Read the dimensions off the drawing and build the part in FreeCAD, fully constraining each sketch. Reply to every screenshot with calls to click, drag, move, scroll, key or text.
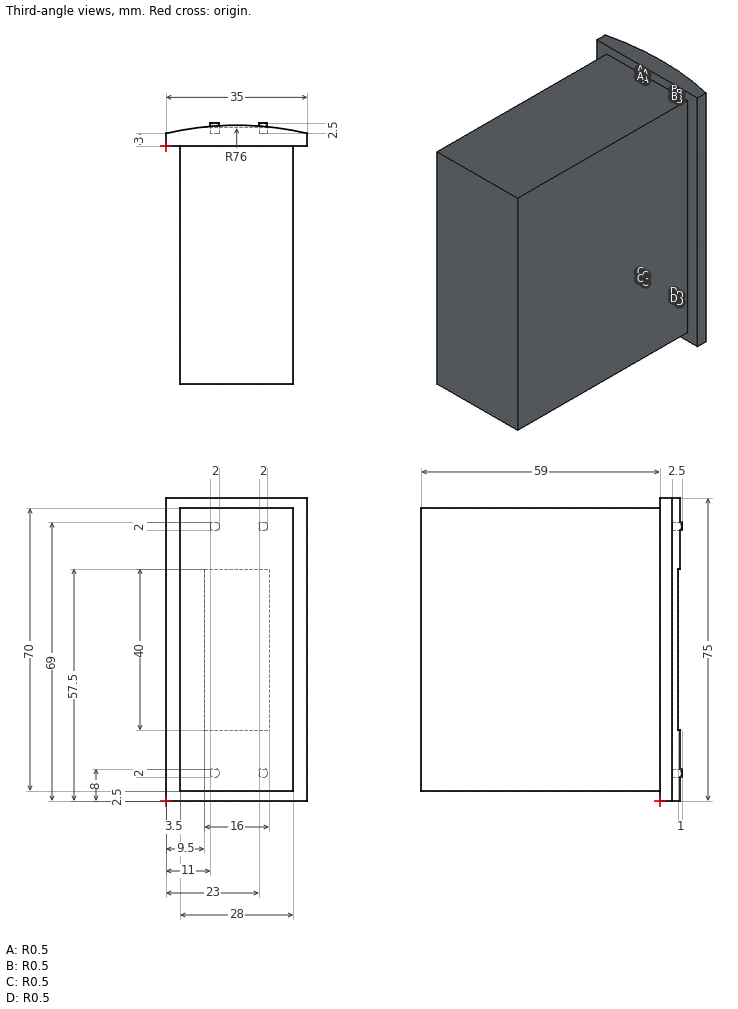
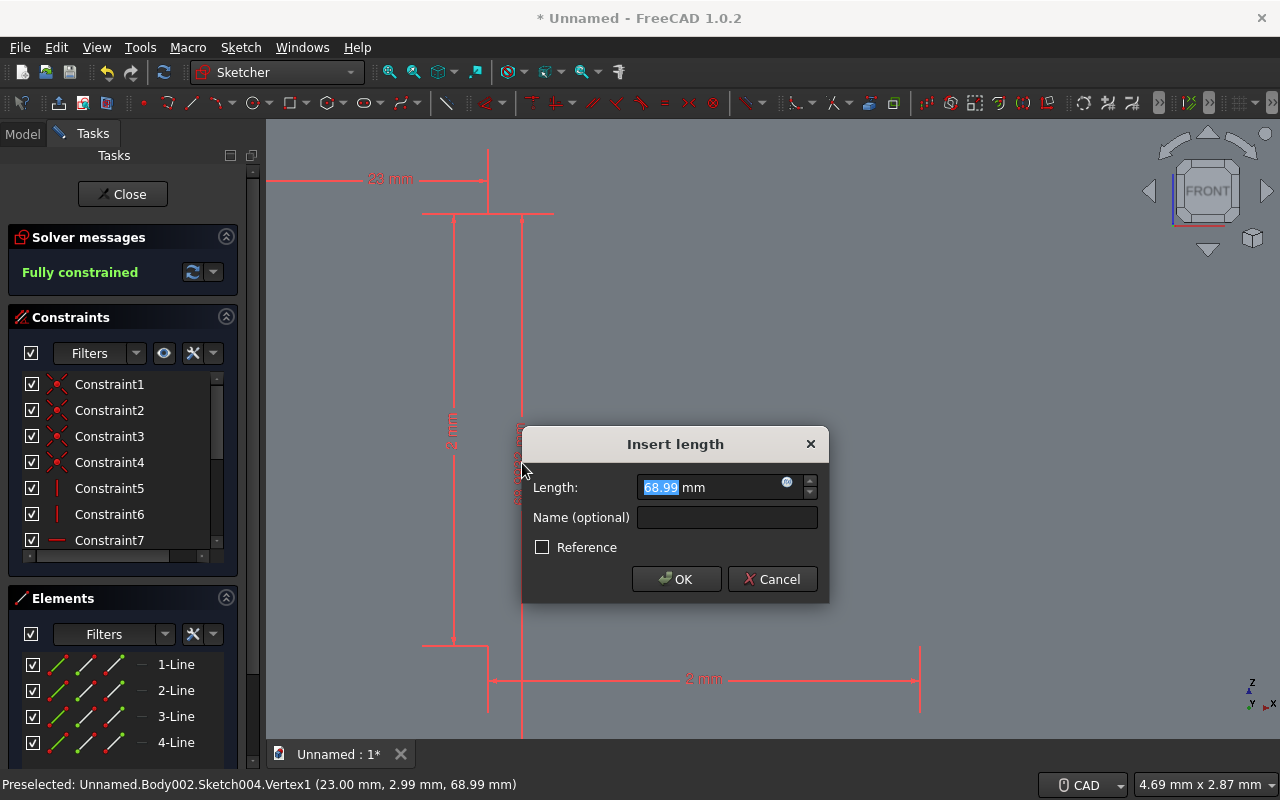
text(69)
key(Return)
key(Escape)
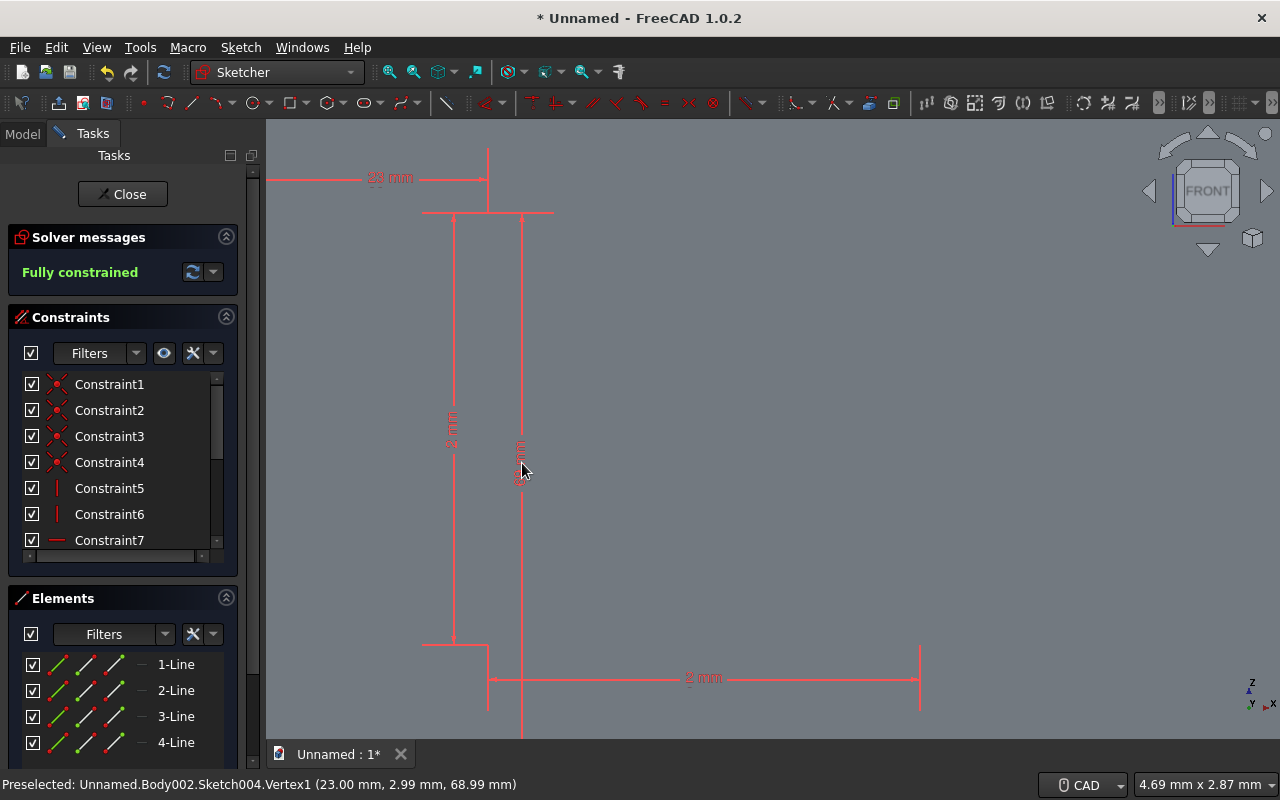
click(123, 194)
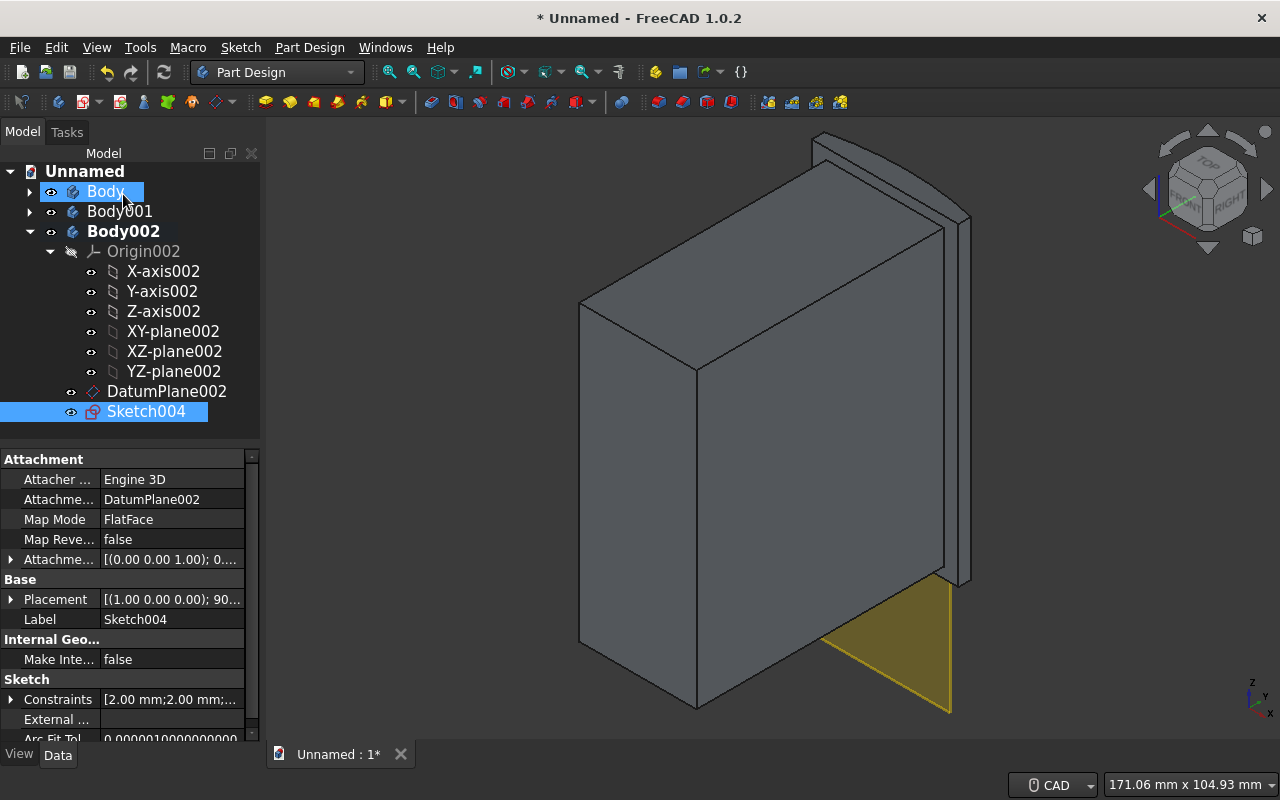
click(266, 102)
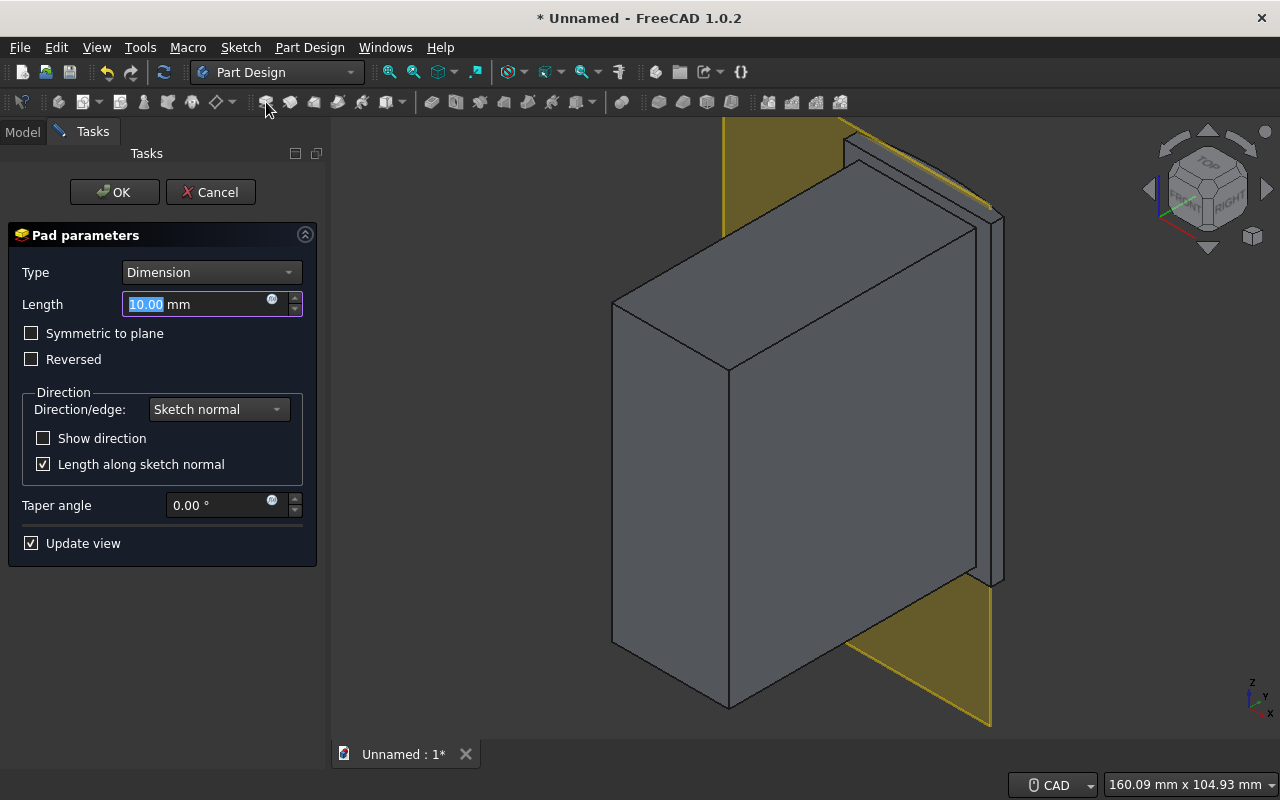
text(2.5)
key(Tab)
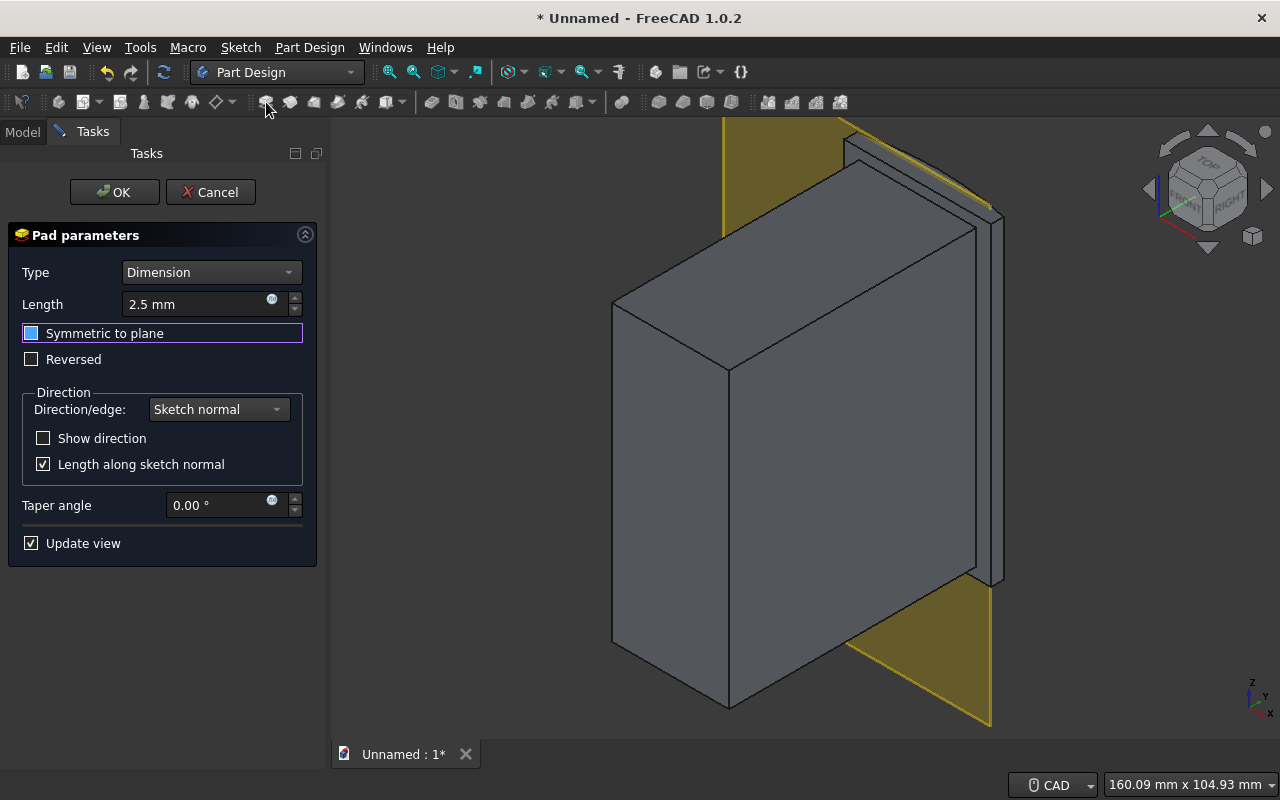
click(30, 359)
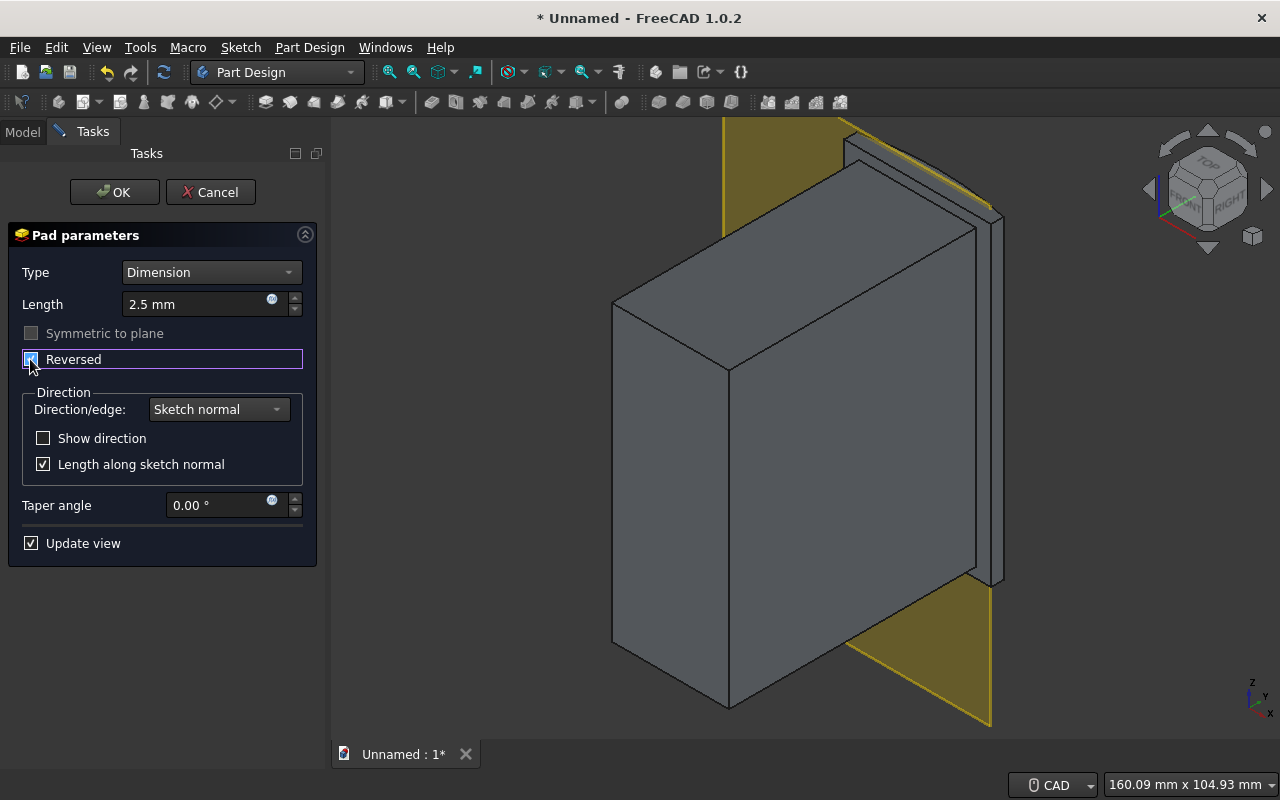
click(115, 192)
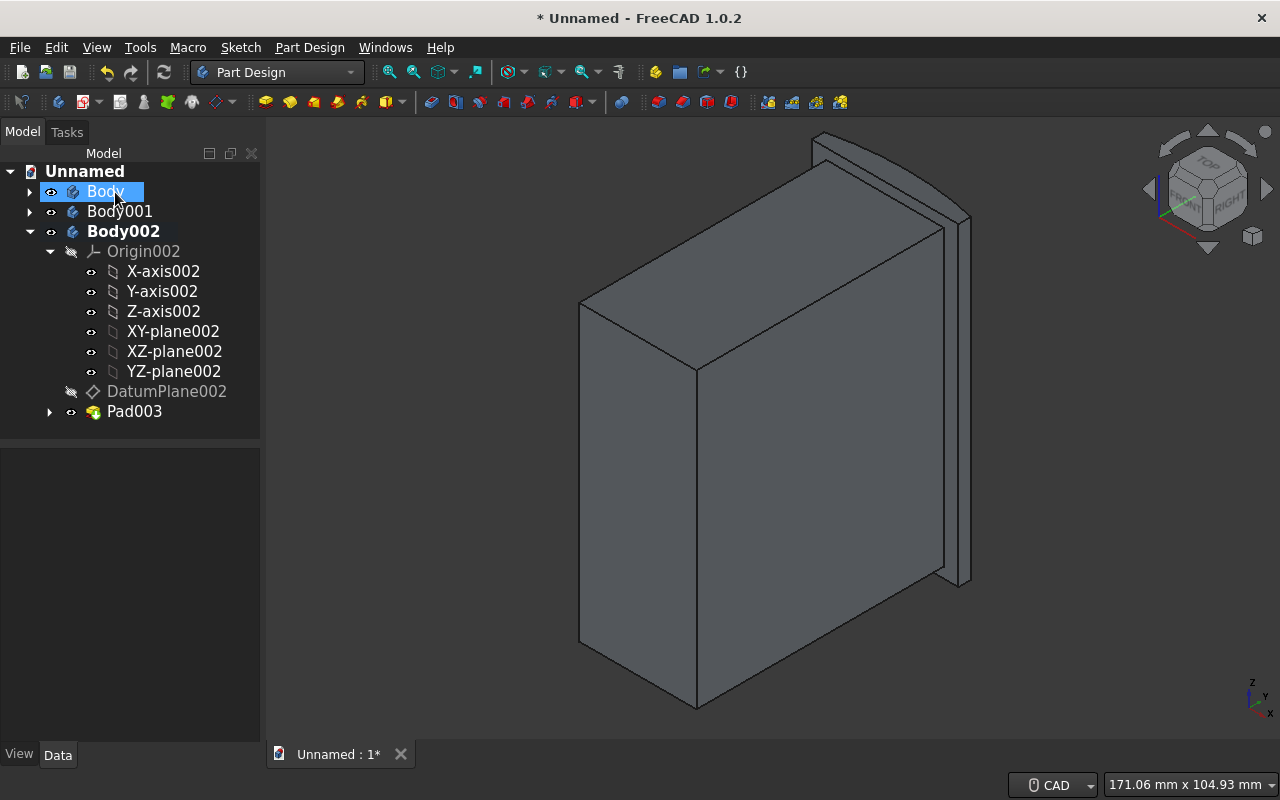
click(390, 72)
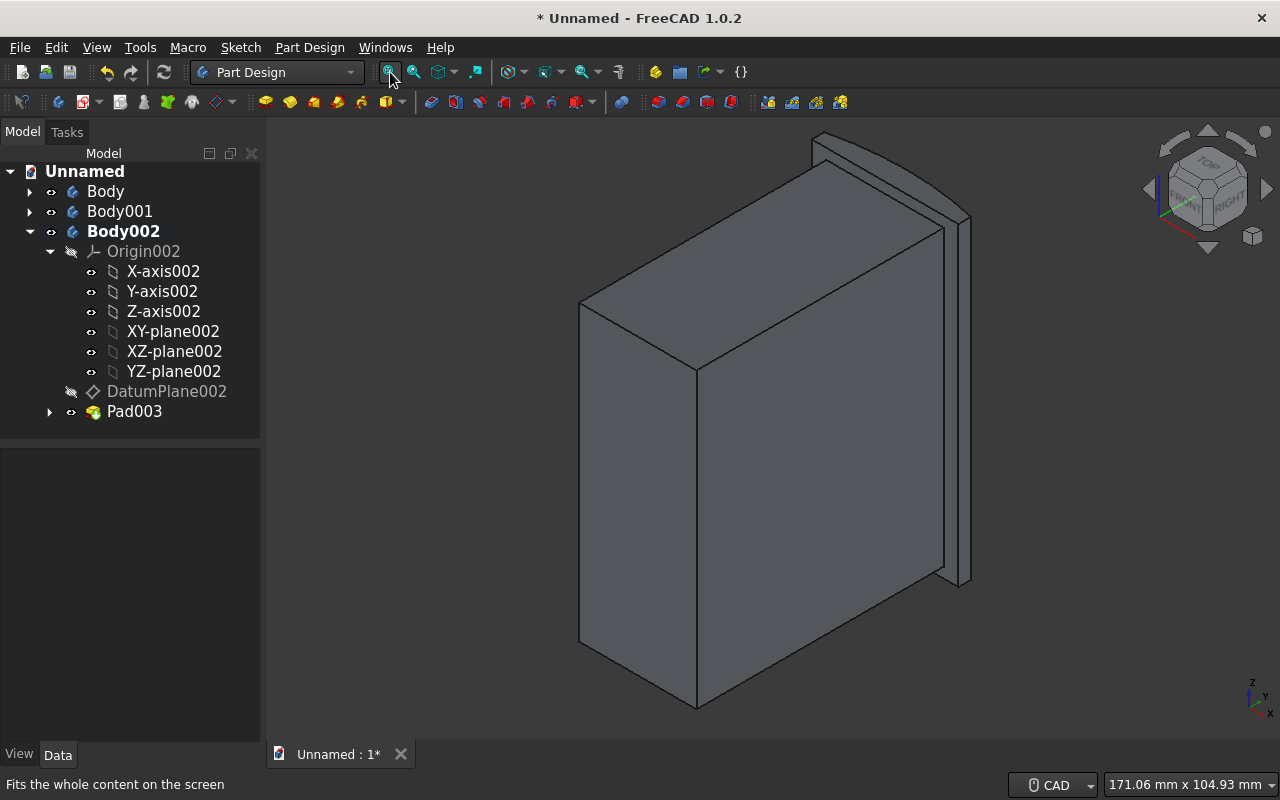
scroll(926, 213, up, 5)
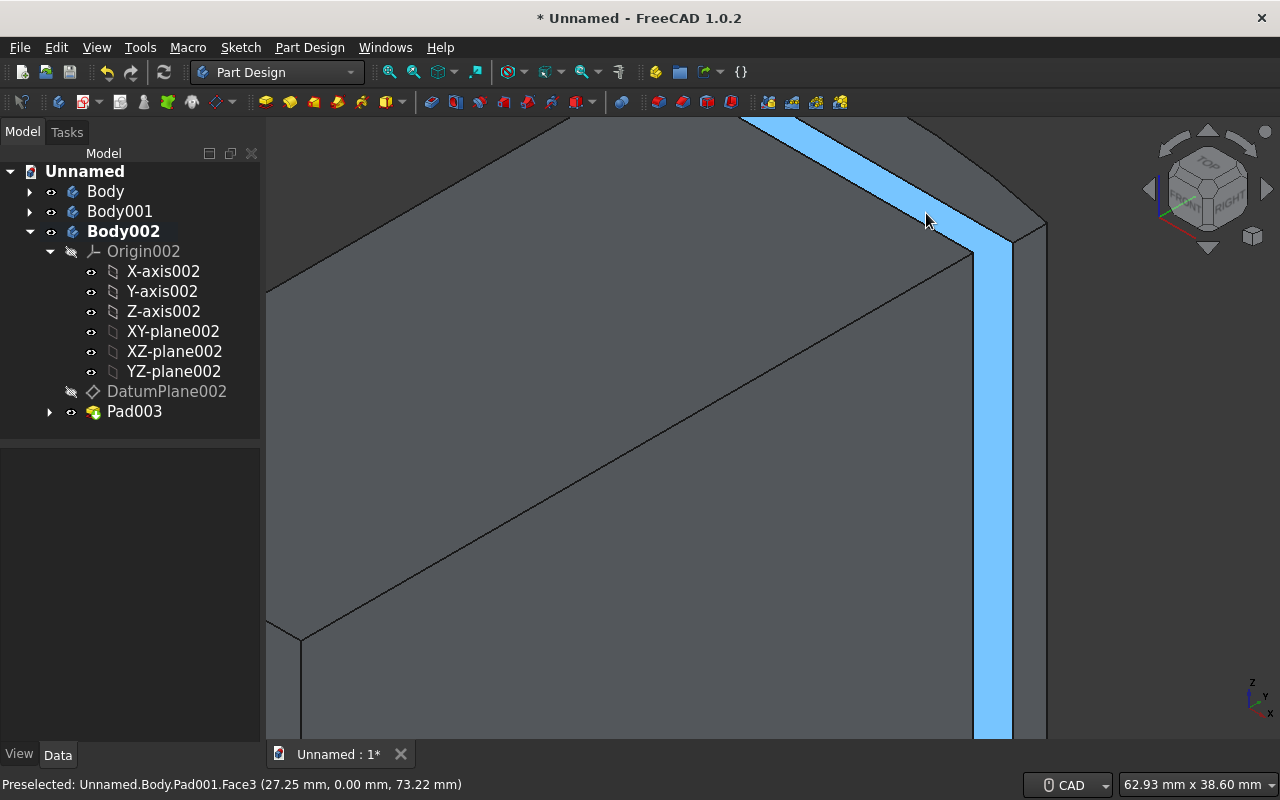
key(v)
key(f)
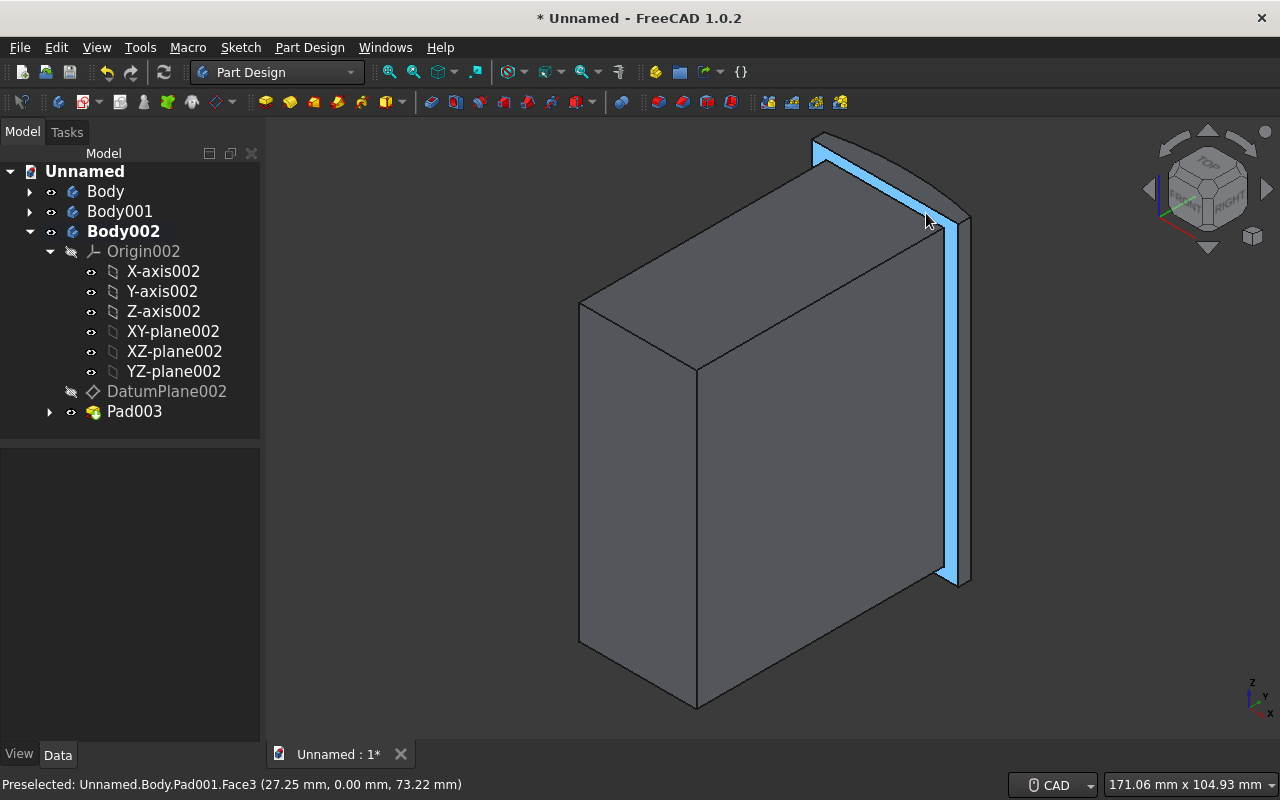
key(2)